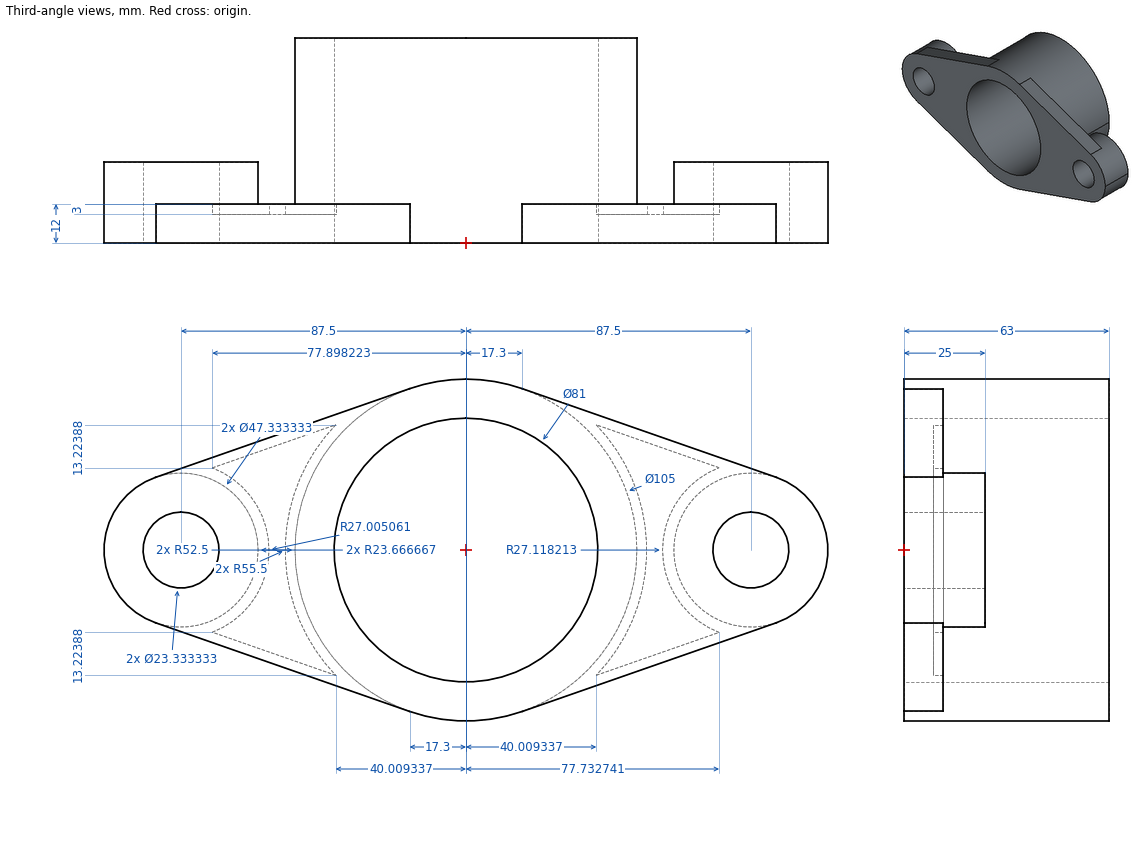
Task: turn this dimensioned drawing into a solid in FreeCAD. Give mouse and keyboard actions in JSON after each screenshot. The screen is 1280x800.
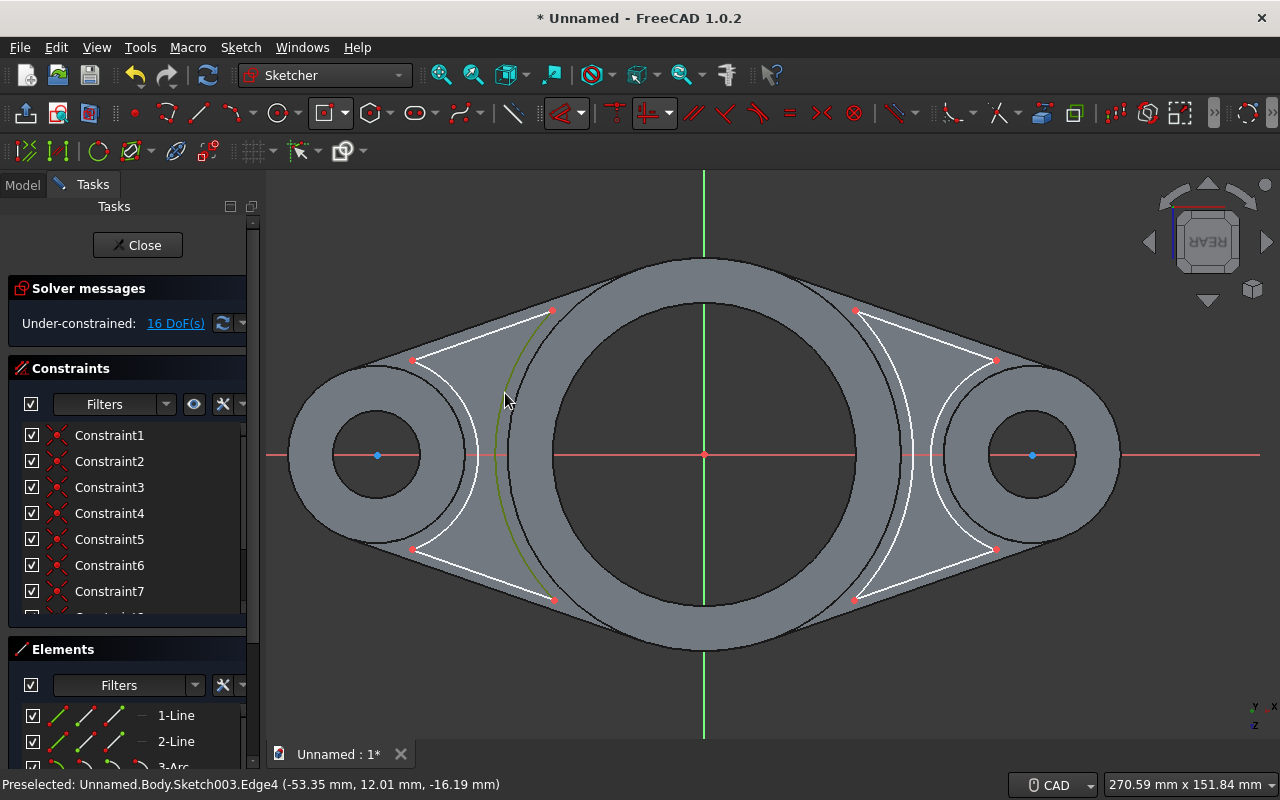
{"action": "left_click", "coordinate": [903, 519]}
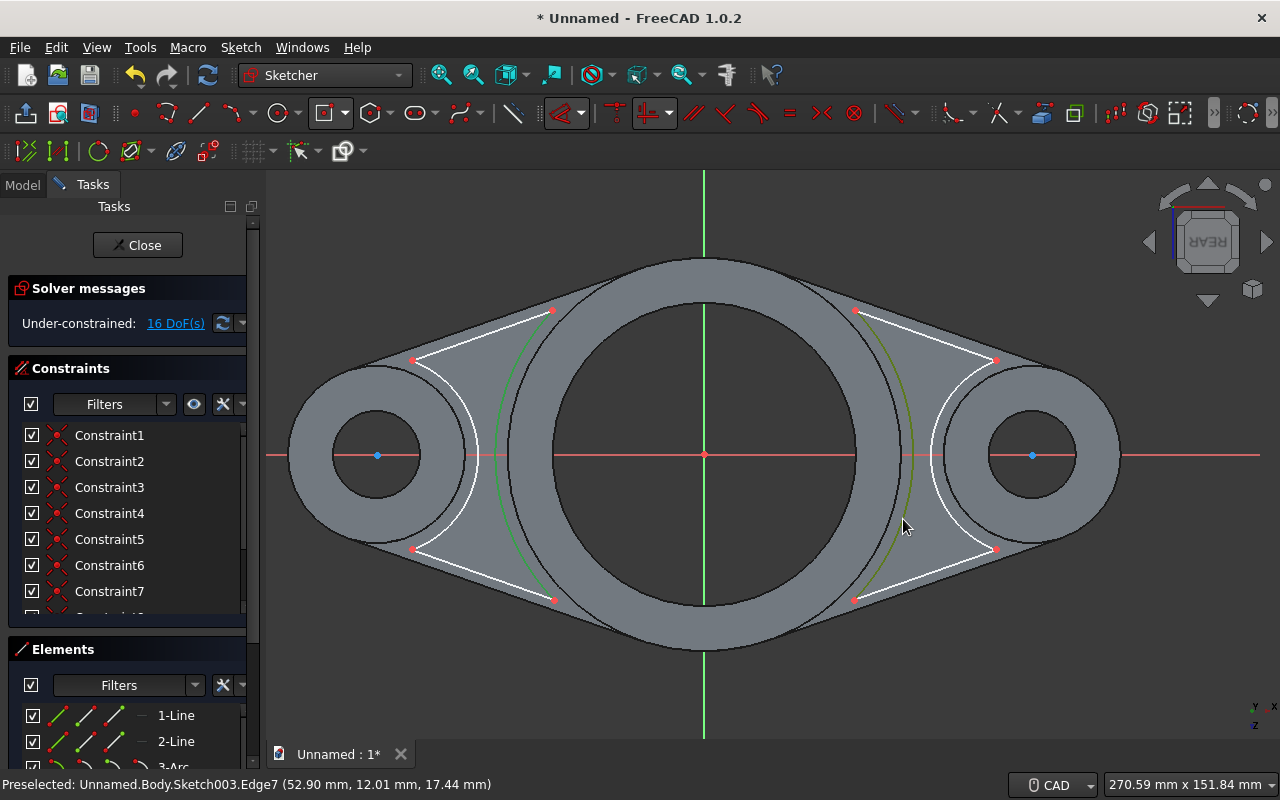
{"action": "key", "text": "e"}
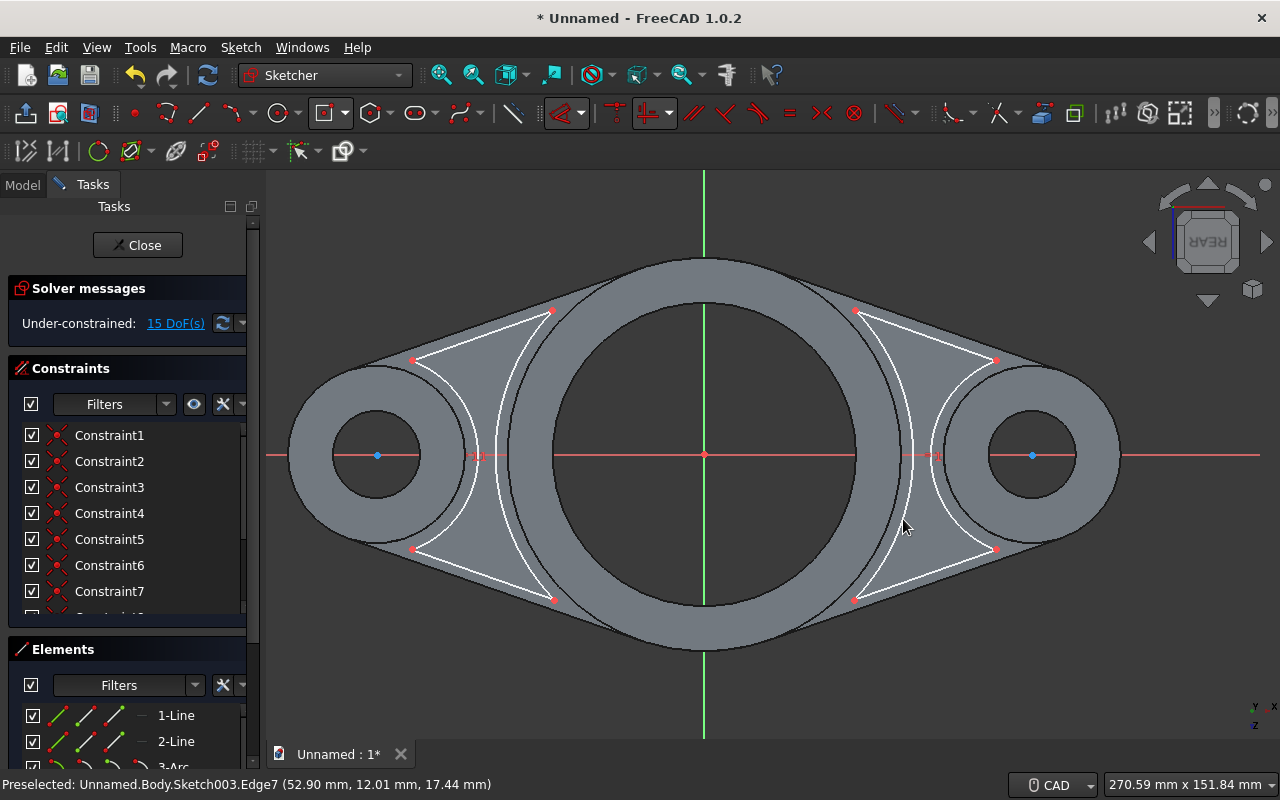
{"action": "left_click", "coordinate": [377, 455]}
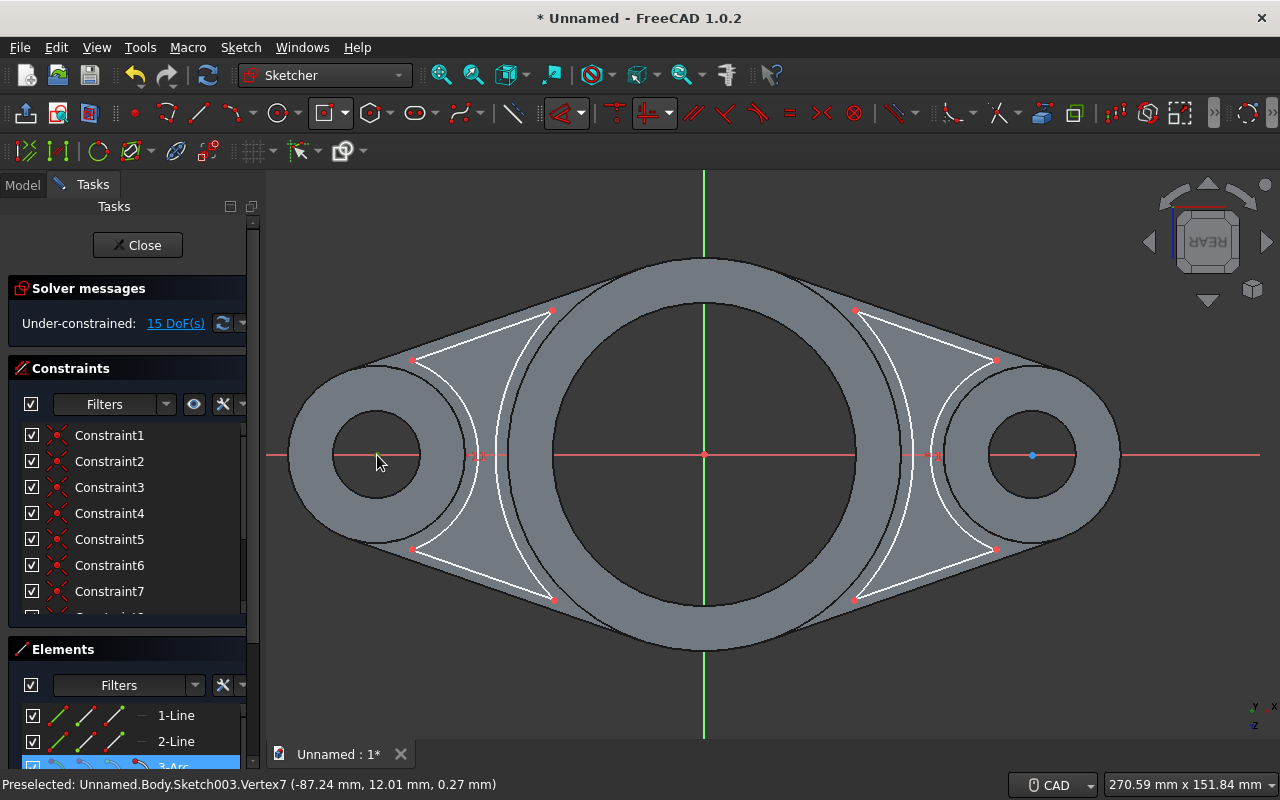
{"action": "left_click", "coordinate": [353, 454]}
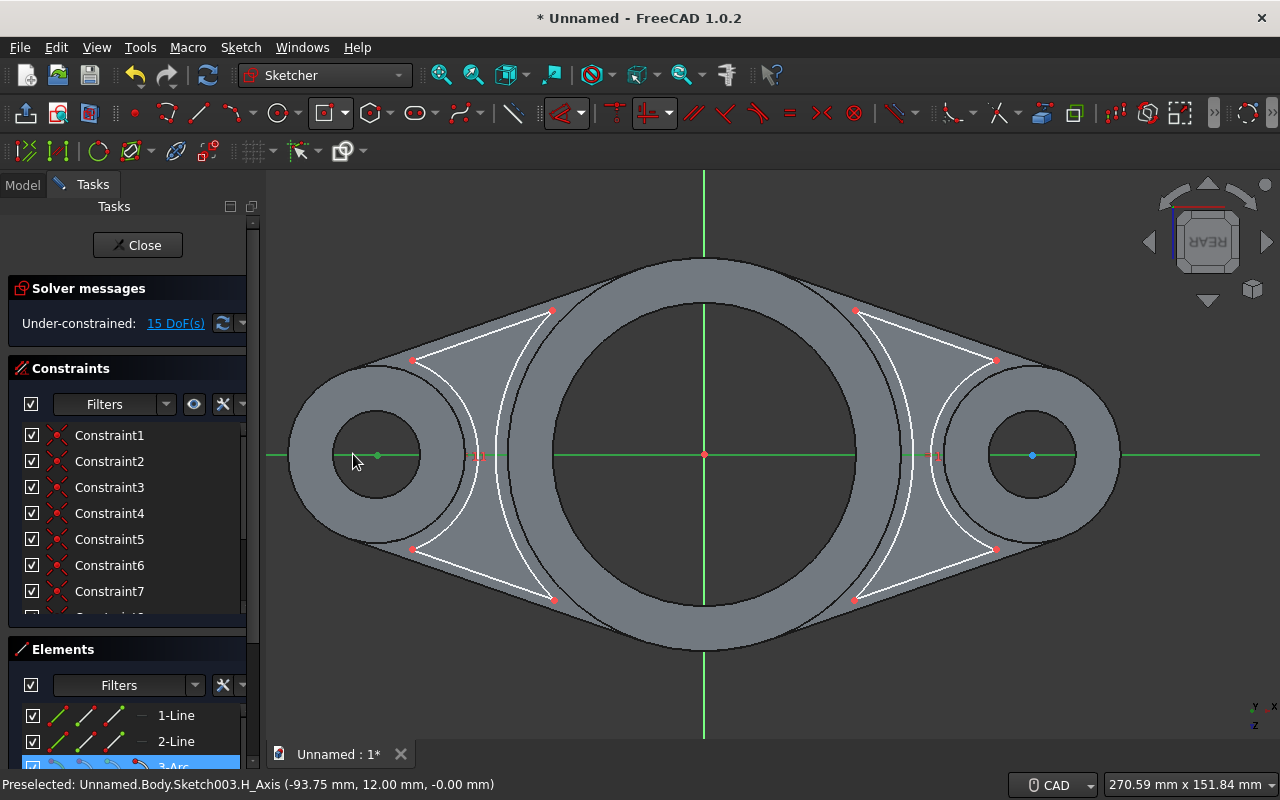
{"action": "key", "text": "c"}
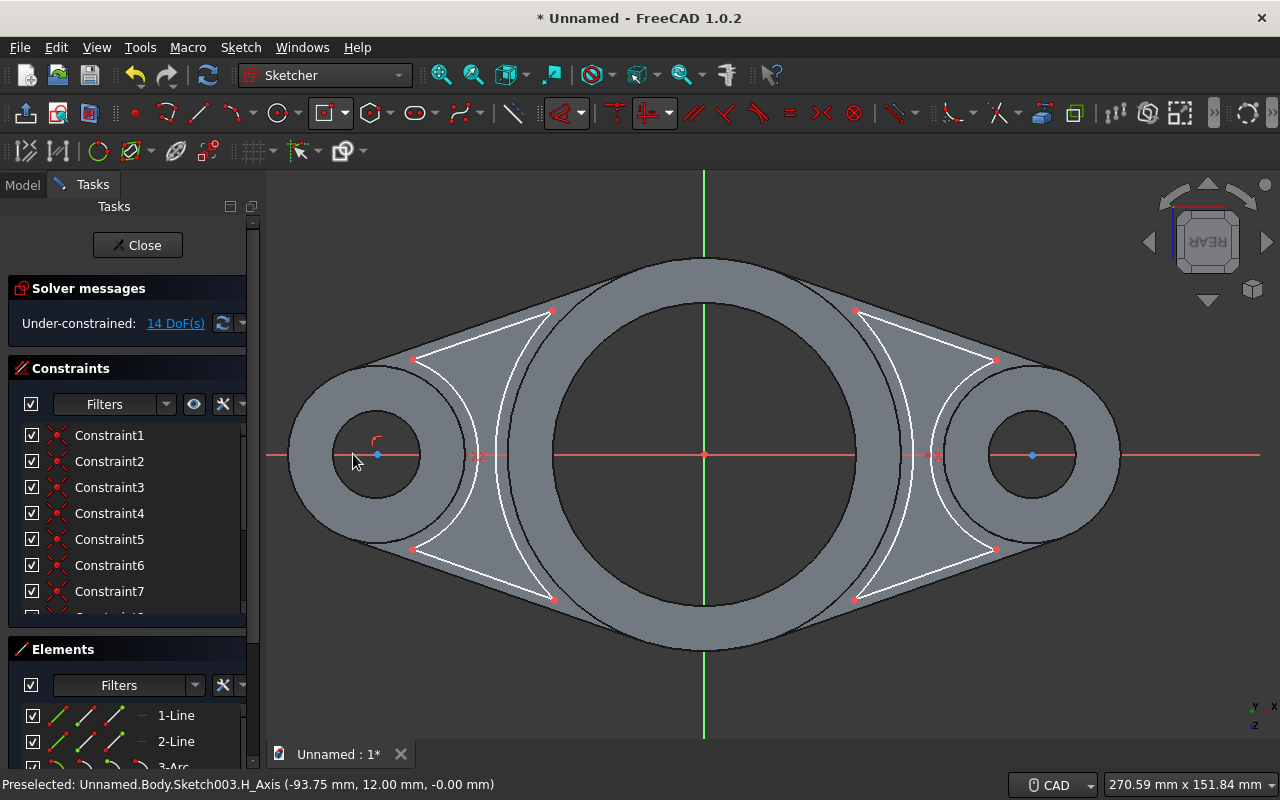
{"action": "left_click", "coordinate": [1032, 455]}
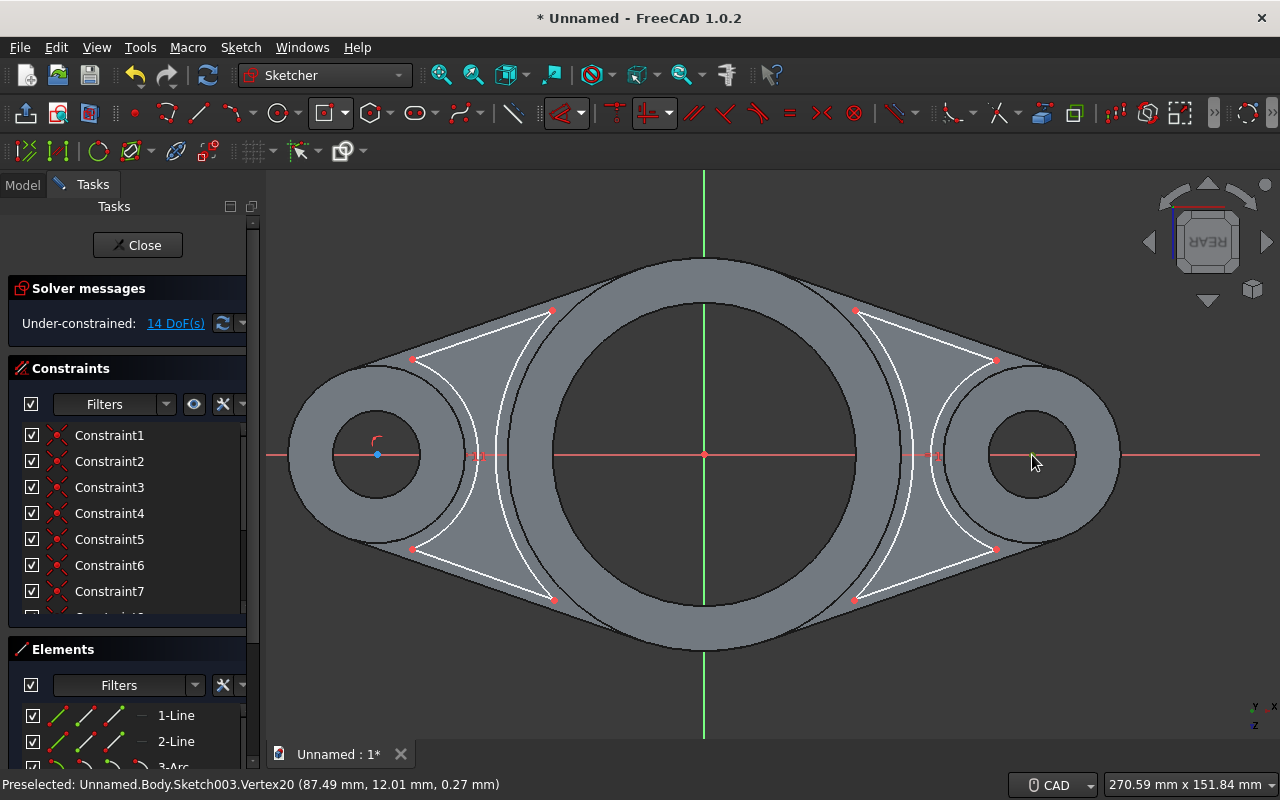
{"action": "left_click", "coordinate": [353, 454]}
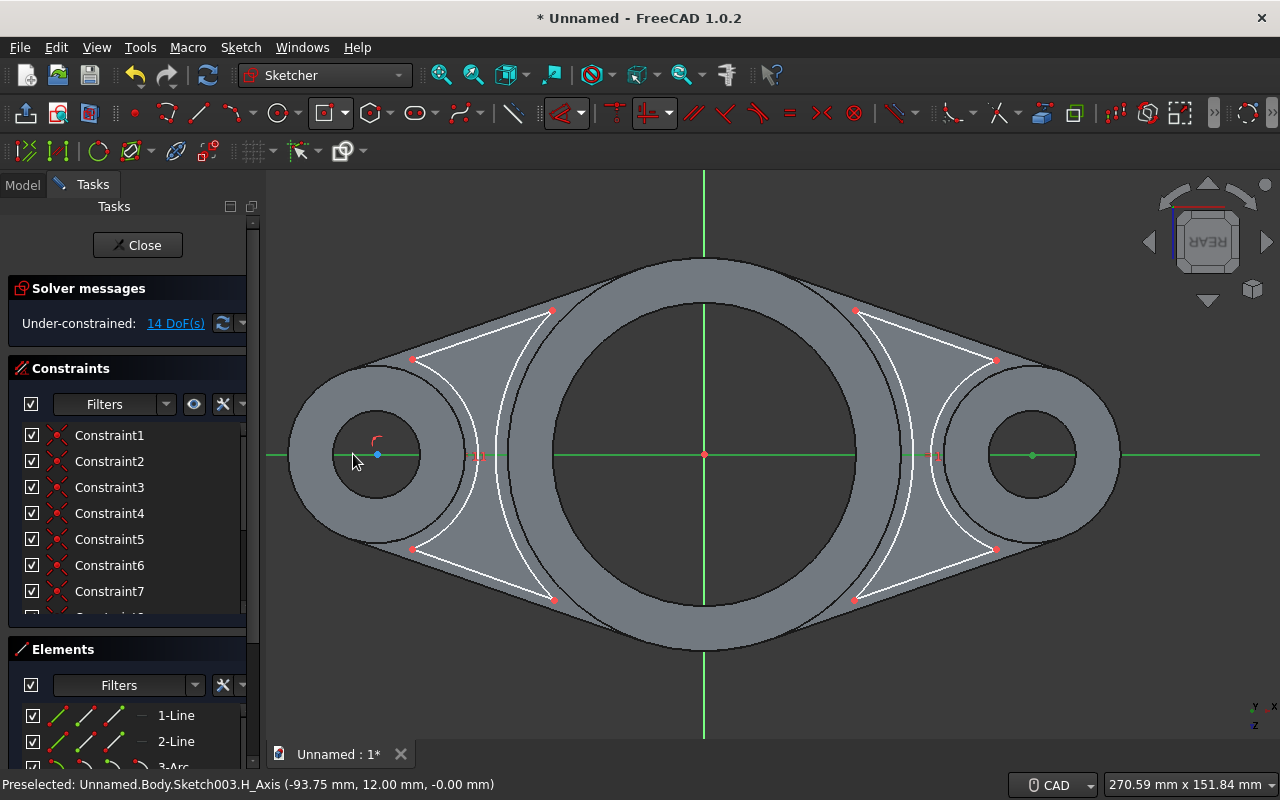
{"action": "key", "text": "c"}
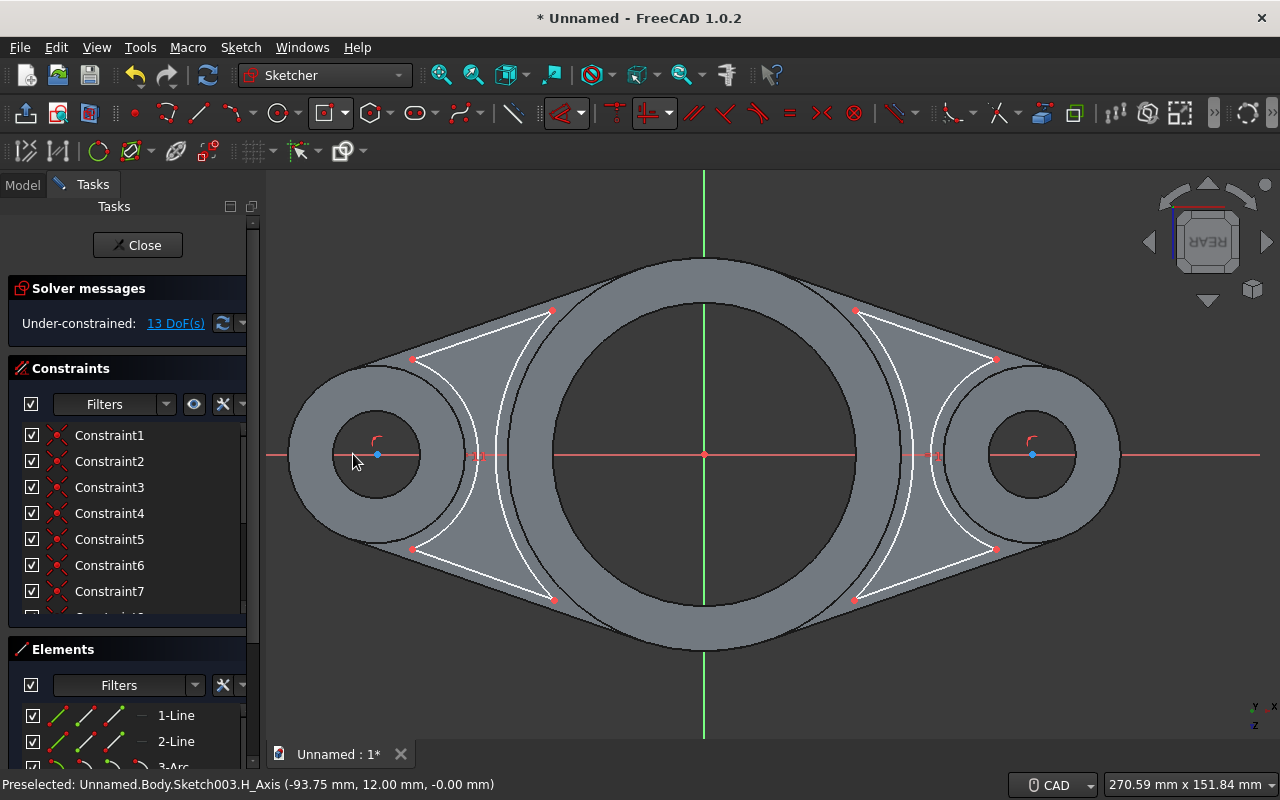
{"action": "left_click", "coordinate": [466, 502]}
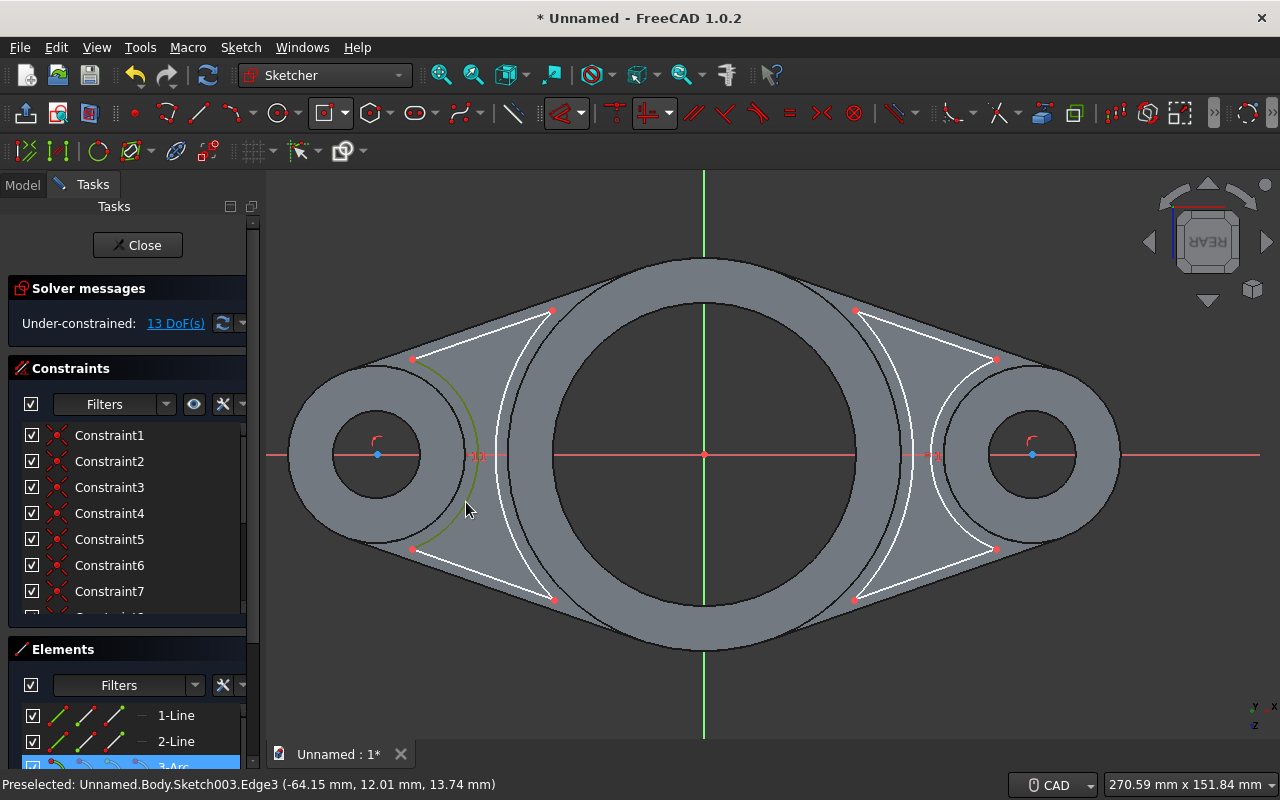
{"action": "key", "text": "k r"}